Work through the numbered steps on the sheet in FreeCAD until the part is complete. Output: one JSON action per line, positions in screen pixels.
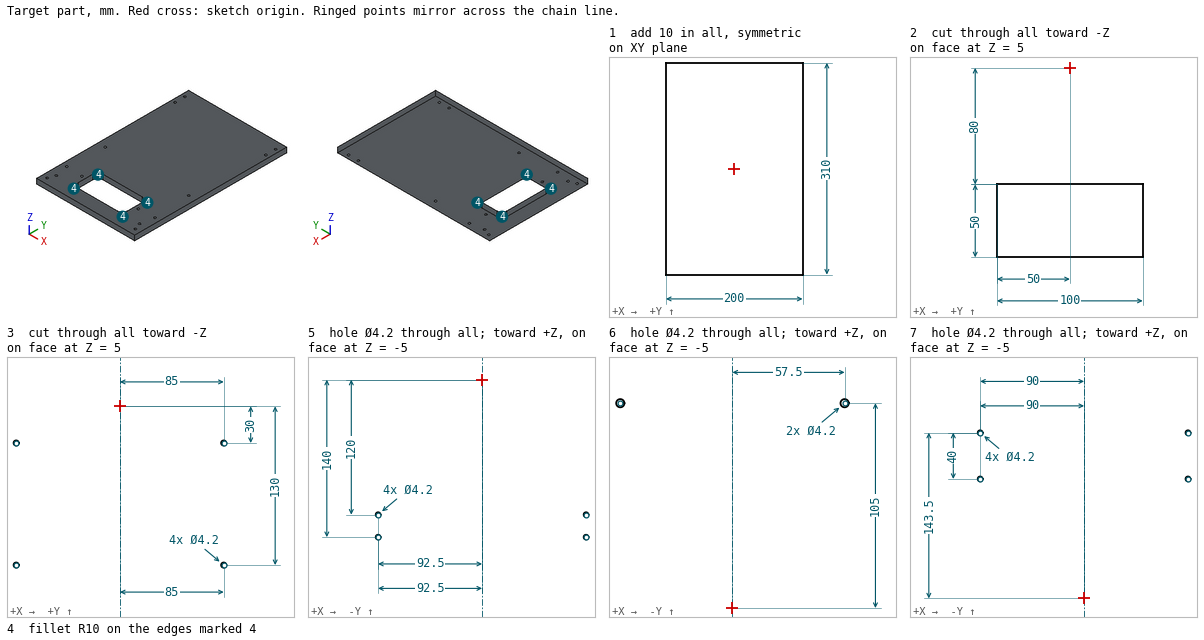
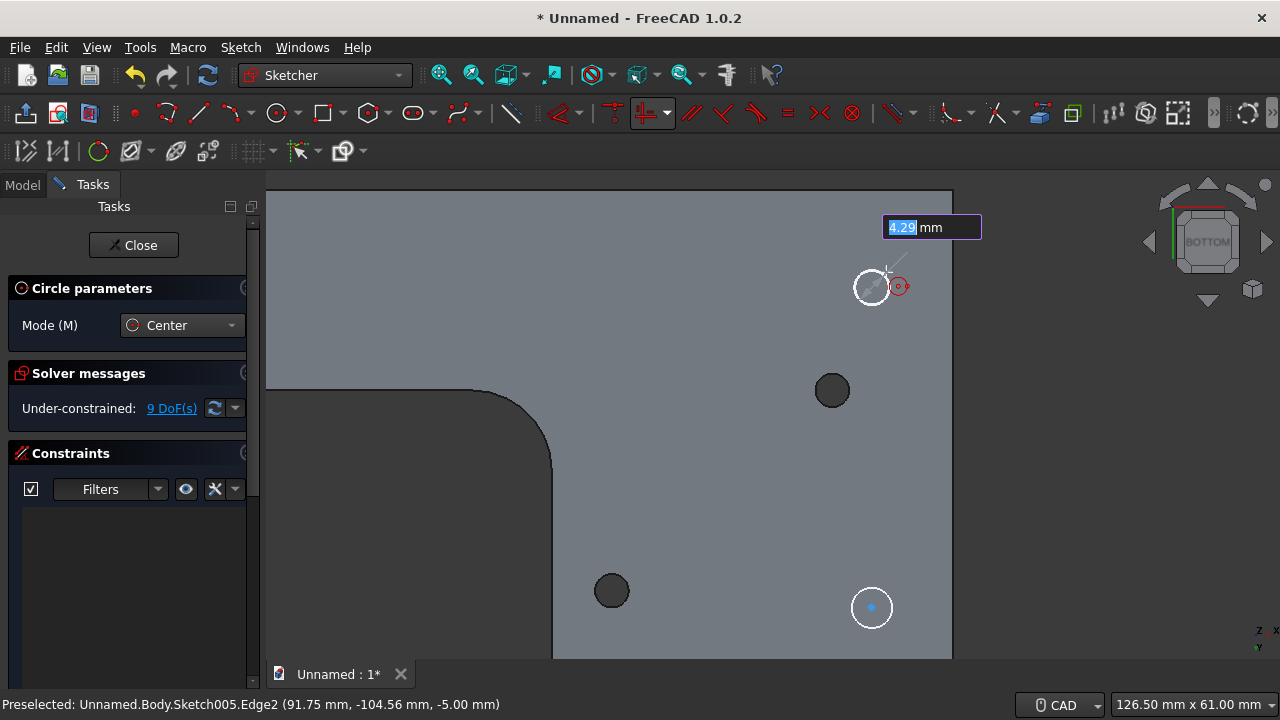
{"action": "left_click", "coordinate": [884, 270]}
{"action": "key", "text": "Escape"}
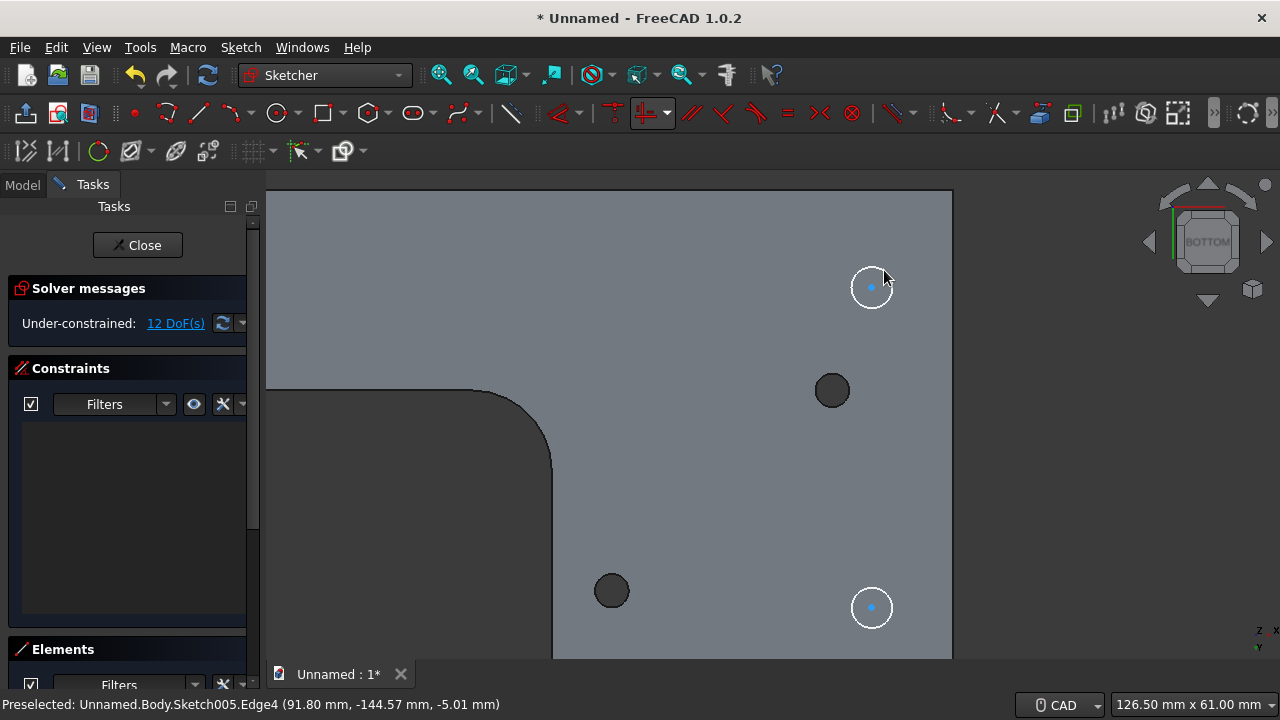
{"action": "scroll", "coordinate": [886, 272], "scroll_direction": "down", "scroll_amount": 7}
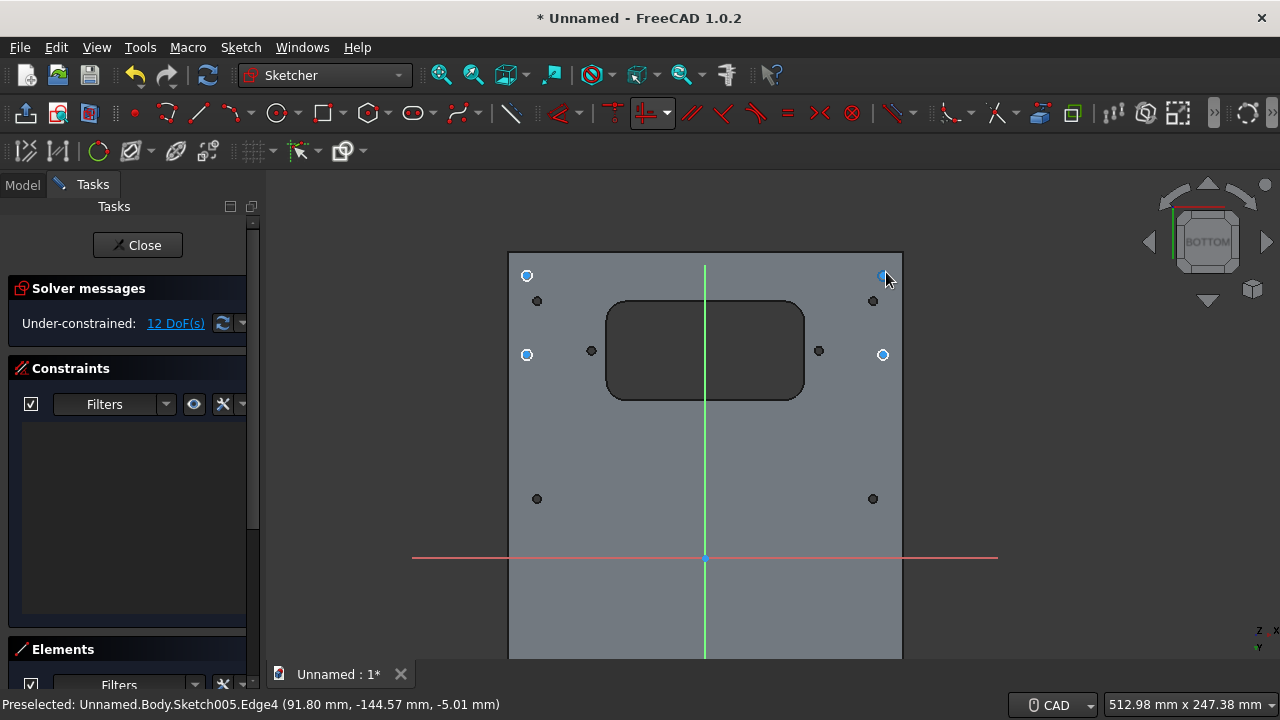
{"action": "scroll", "coordinate": [531, 272], "scroll_direction": "up", "scroll_amount": 5}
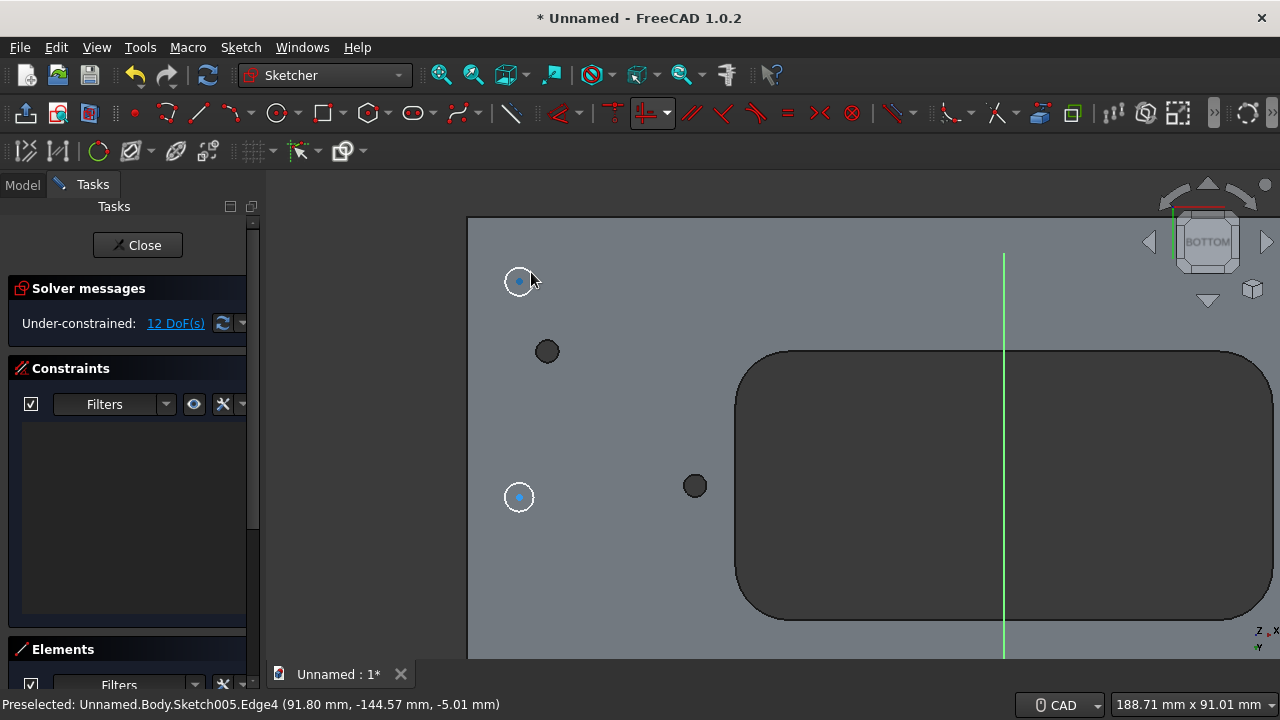
{"action": "left_click", "coordinate": [529, 272]}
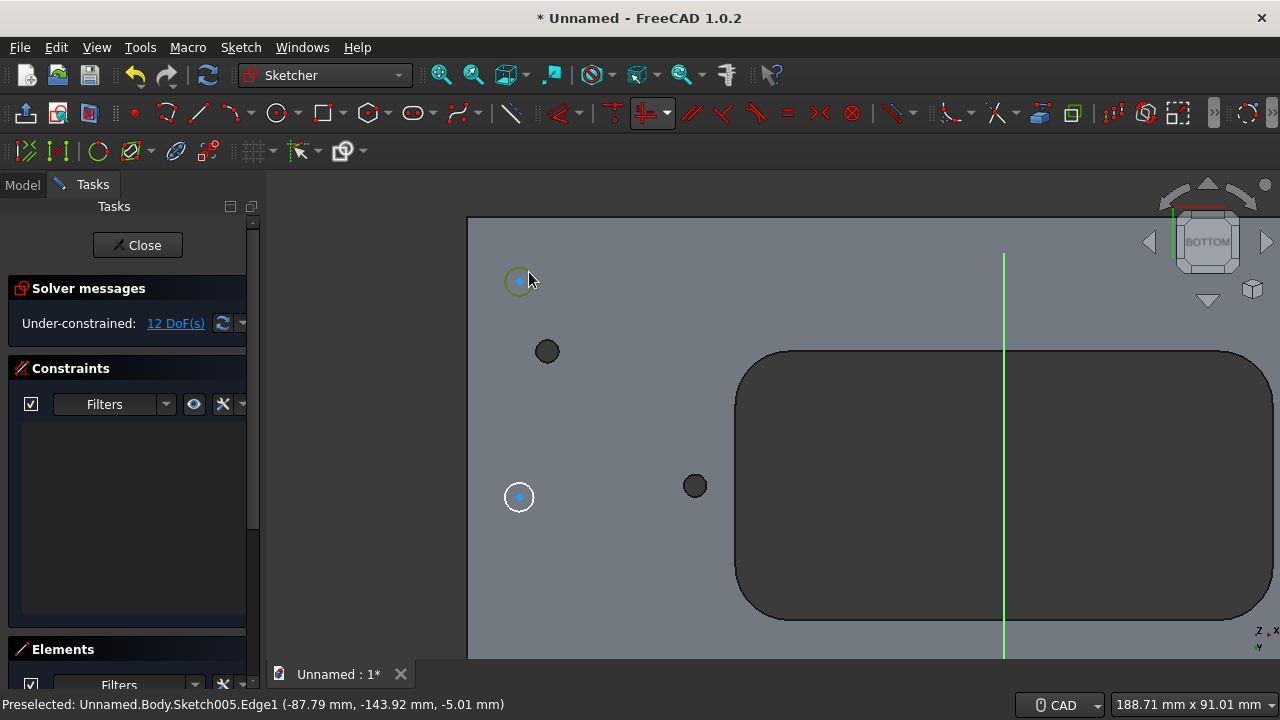
{"action": "left_click", "coordinate": [529, 487]}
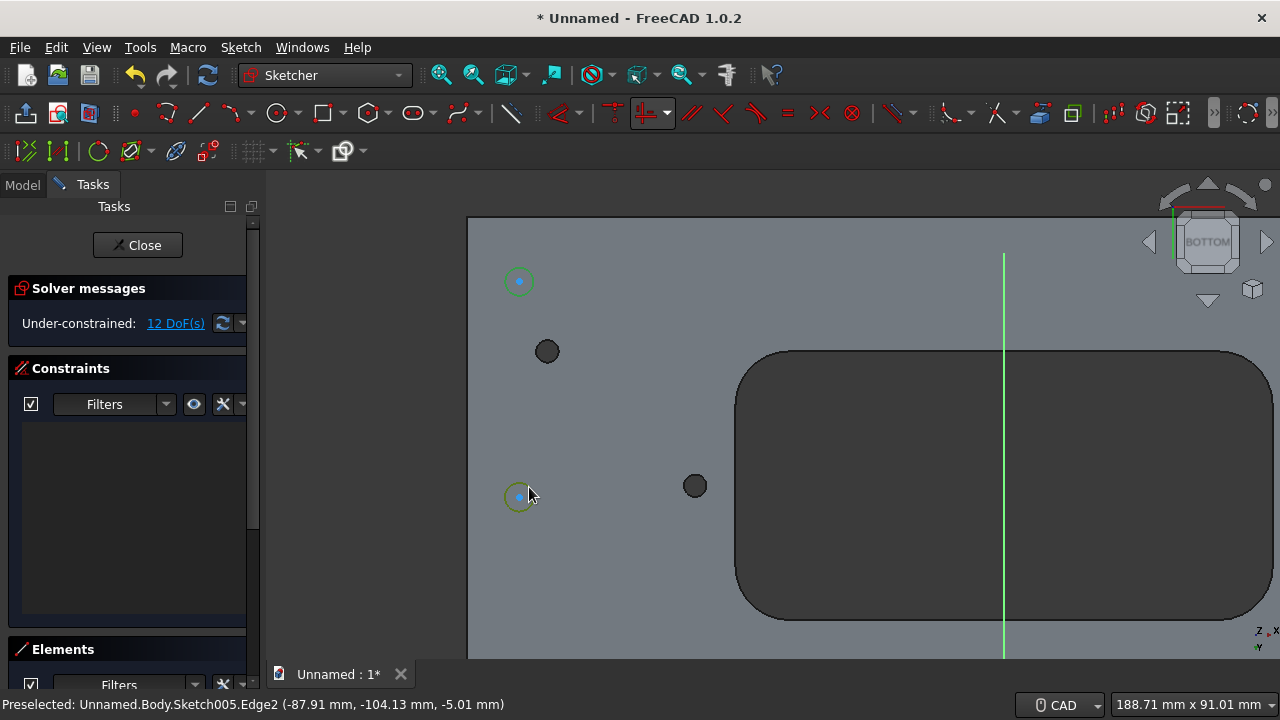
{"action": "scroll", "coordinate": [530, 272], "scroll_direction": "down", "scroll_amount": 5}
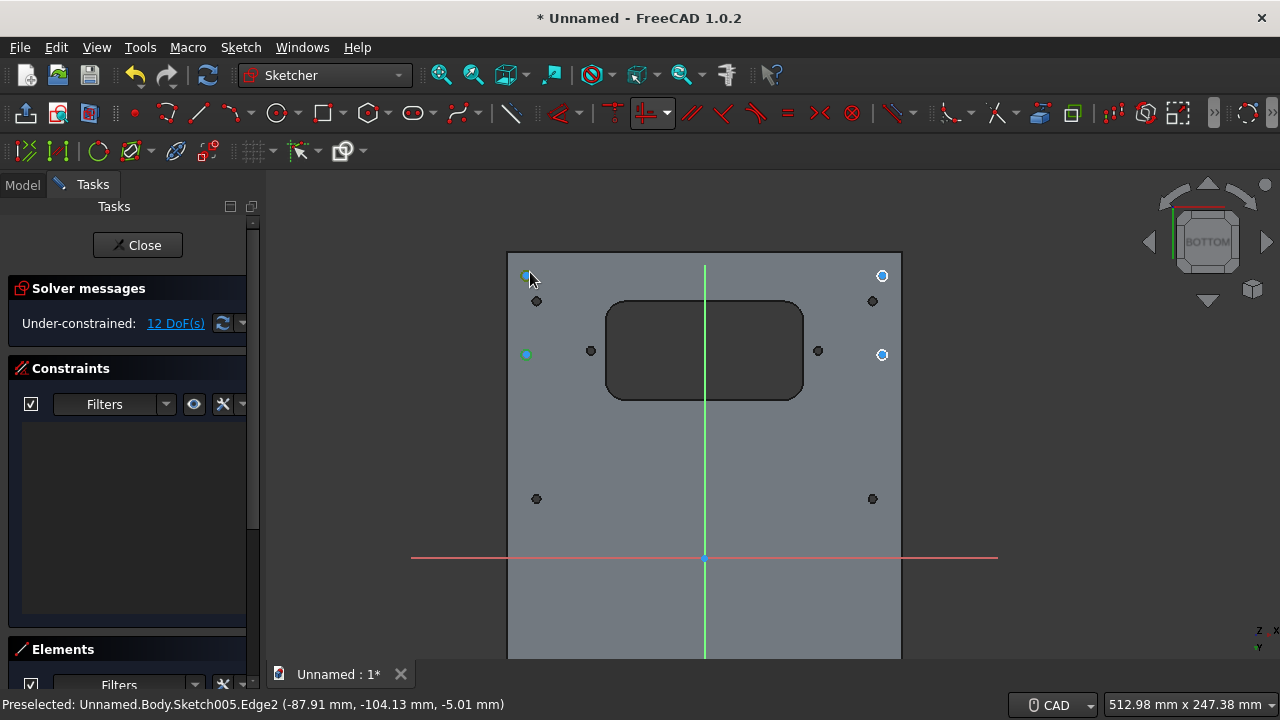
{"action": "scroll", "coordinate": [886, 351], "scroll_direction": "up", "scroll_amount": 6}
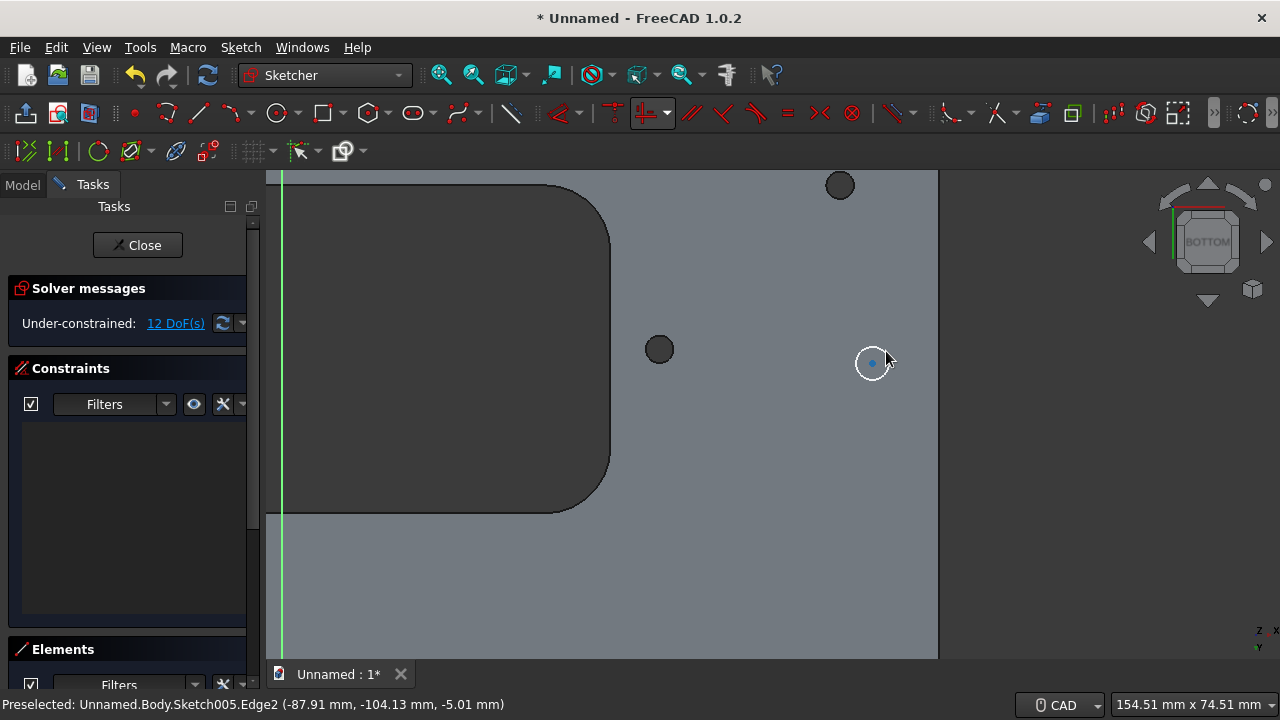
{"action": "left_click", "coordinate": [884, 352]}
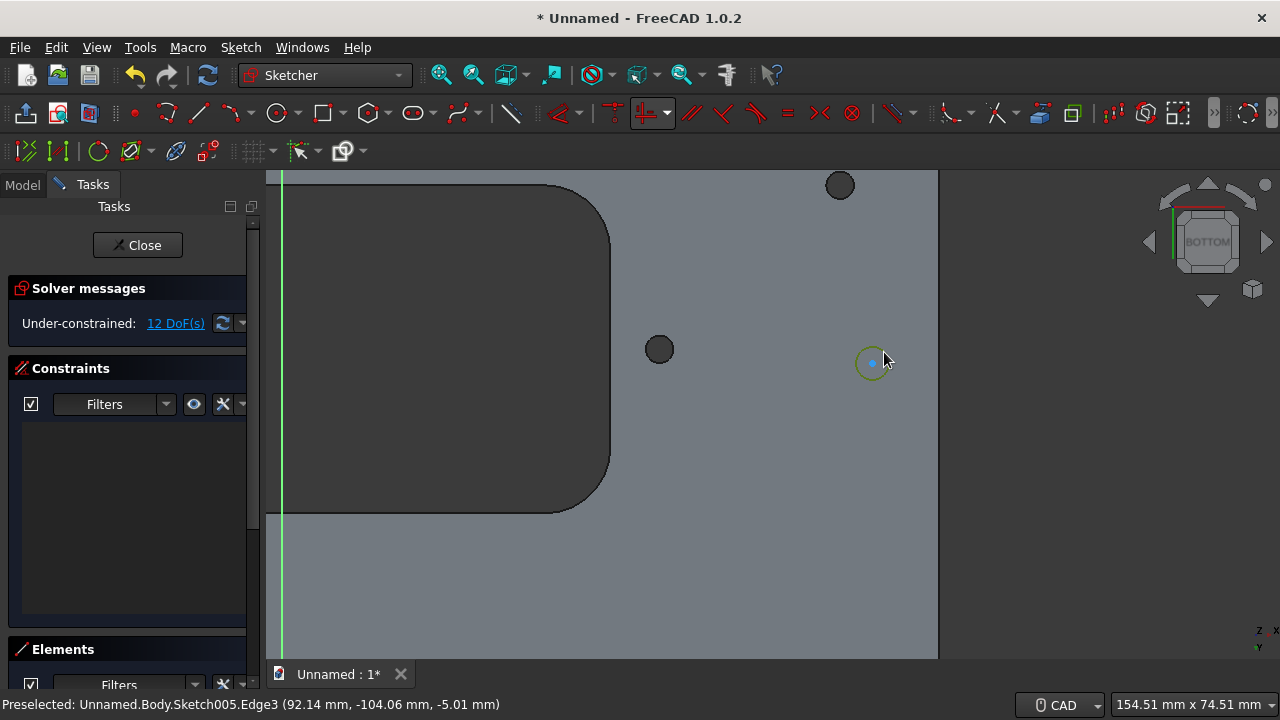
{"action": "scroll", "coordinate": [886, 352], "scroll_direction": "down", "scroll_amount": 6}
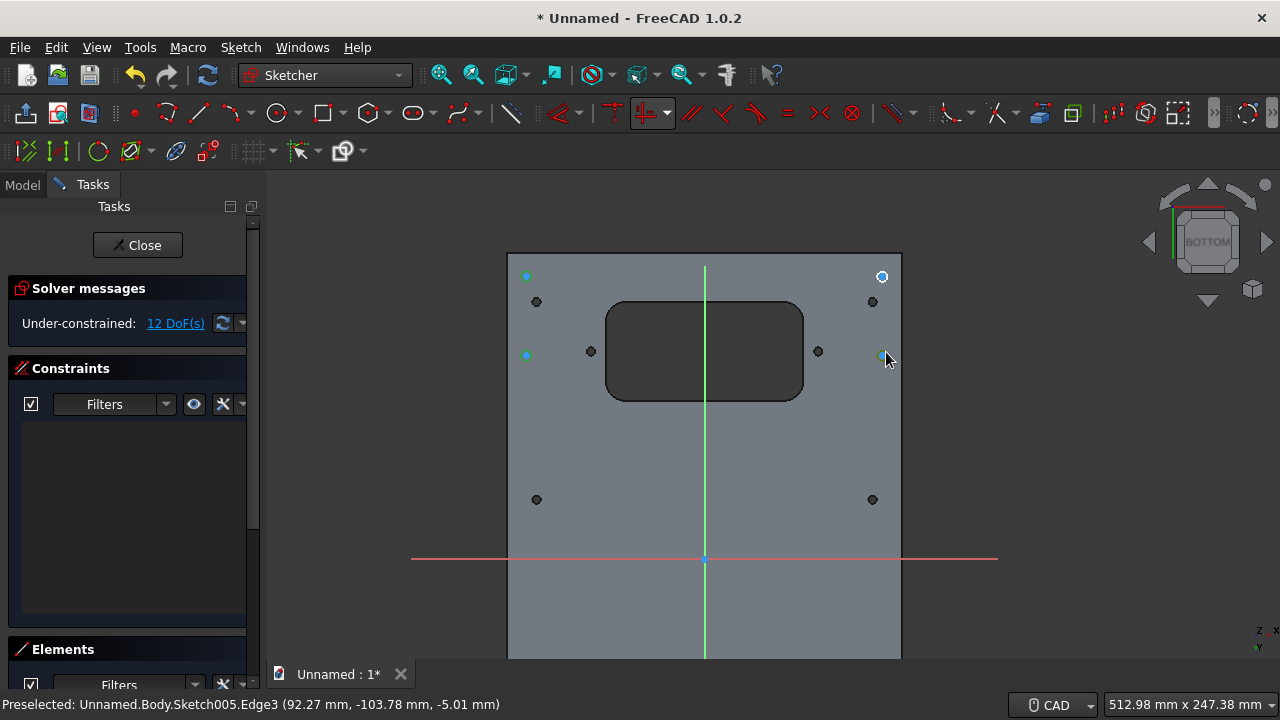
{"action": "scroll", "coordinate": [886, 273], "scroll_direction": "up", "scroll_amount": 6}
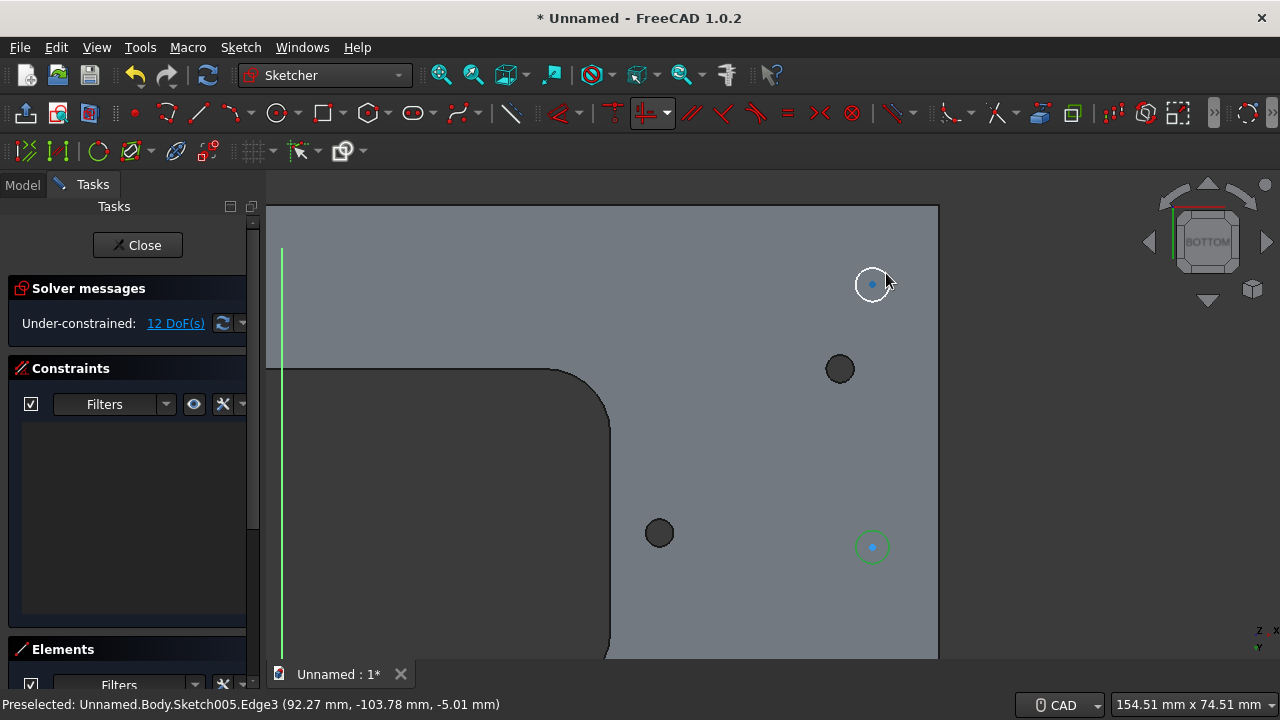
{"action": "left_click", "coordinate": [884, 273]}